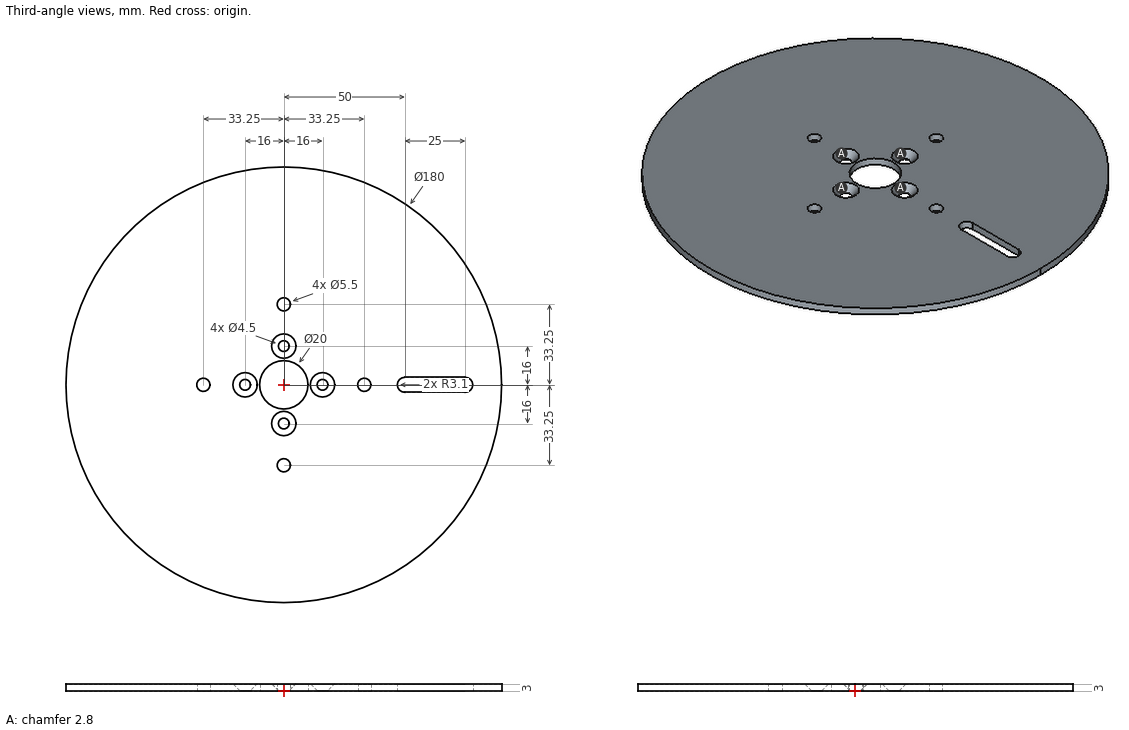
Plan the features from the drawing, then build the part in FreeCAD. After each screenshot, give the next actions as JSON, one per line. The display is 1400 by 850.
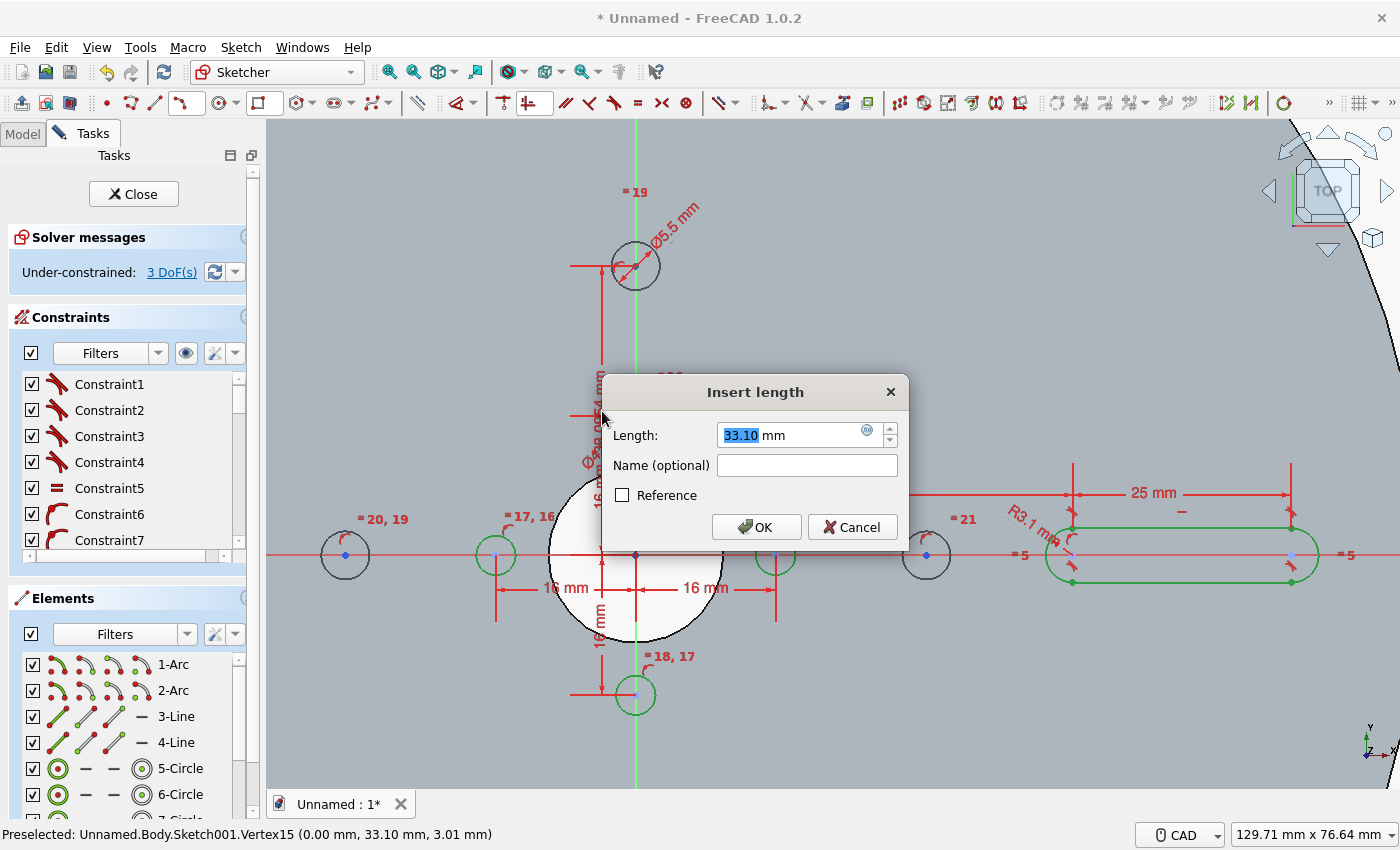
{"action": "type", "text": "33.25"}
{"action": "key", "text": "Return"}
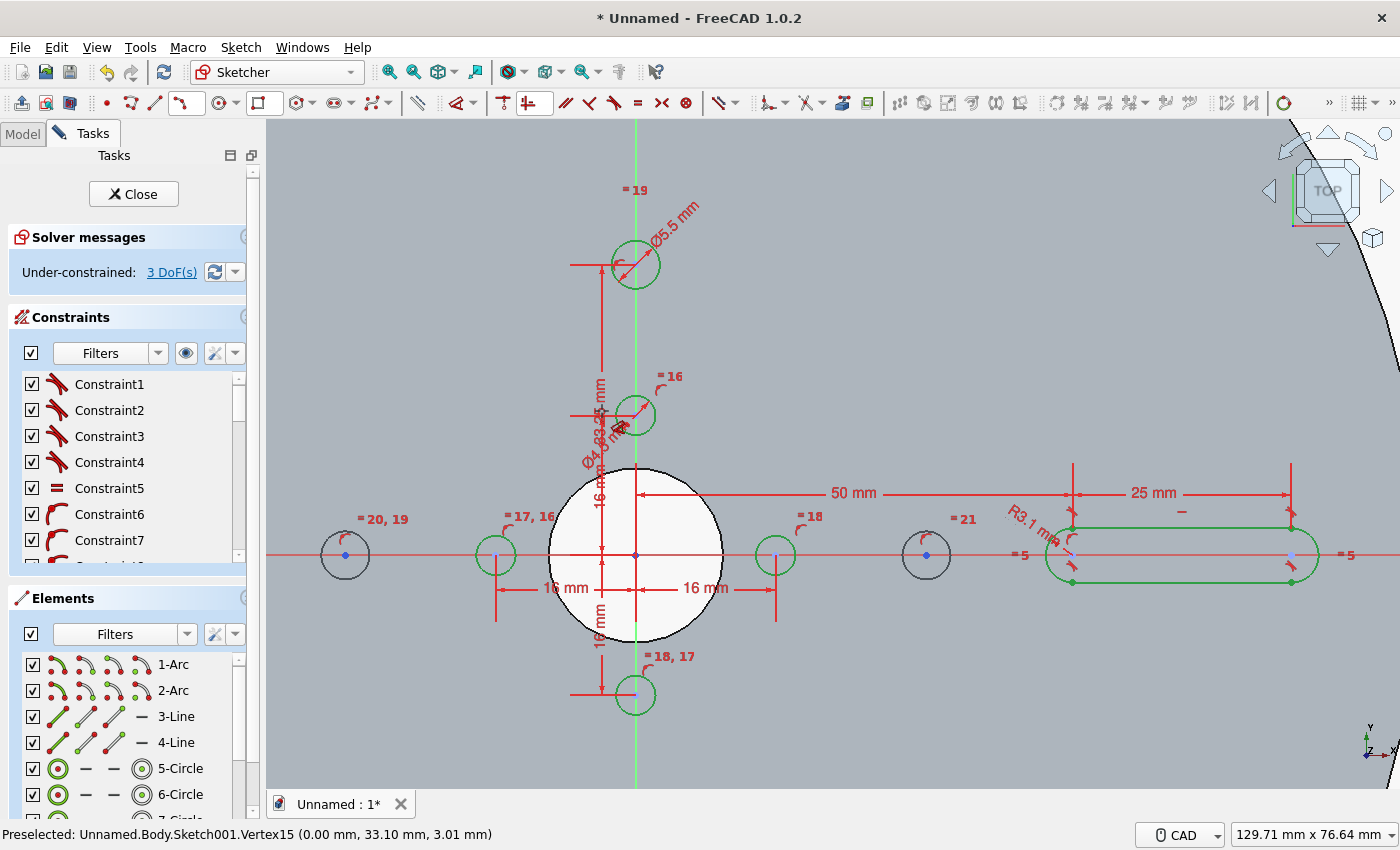
{"action": "left_click", "coordinate": [345, 555]}
{"action": "left_click", "coordinate": [491, 589]}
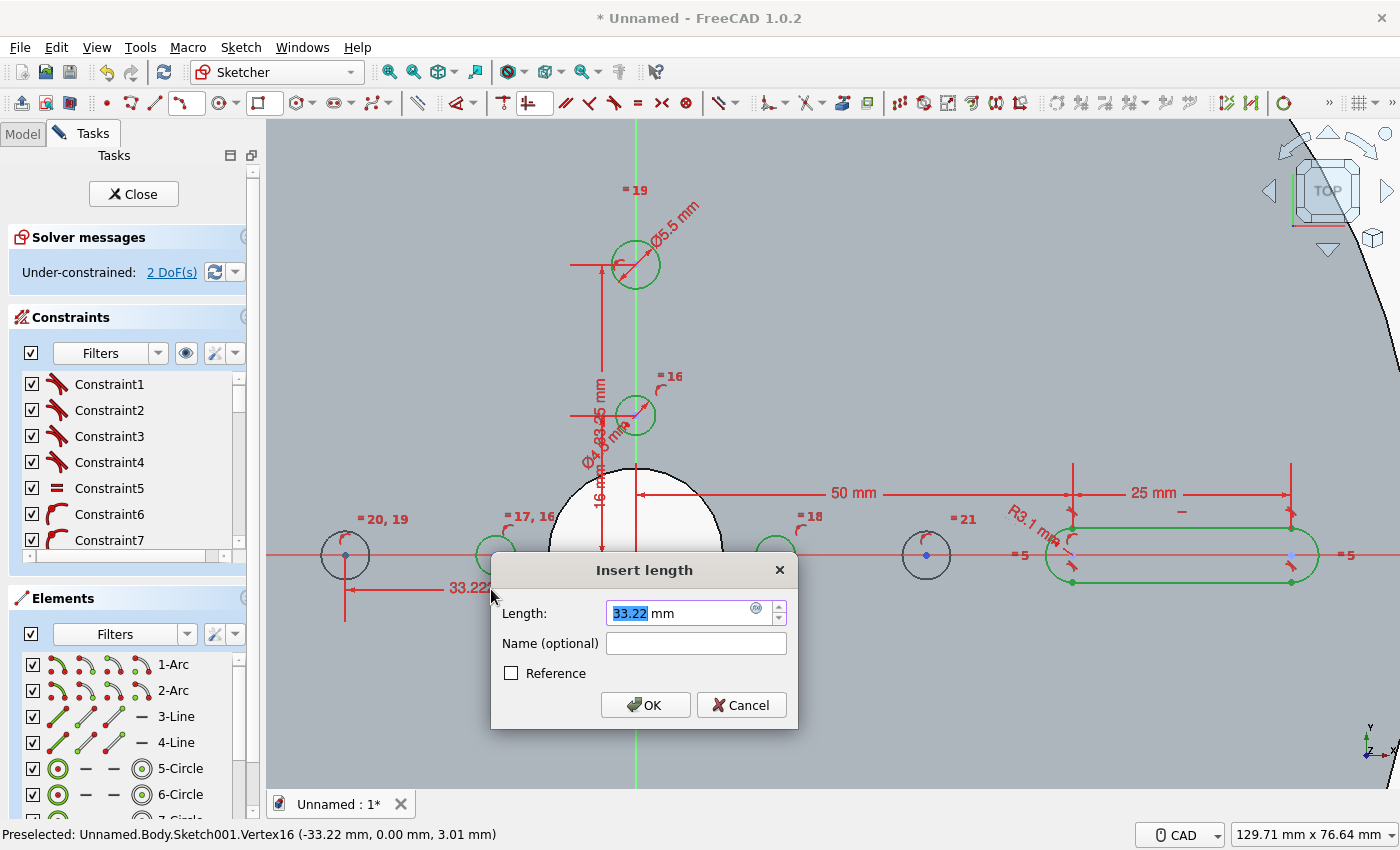
{"action": "type", "text": "33.25"}
{"action": "key", "text": "Return"}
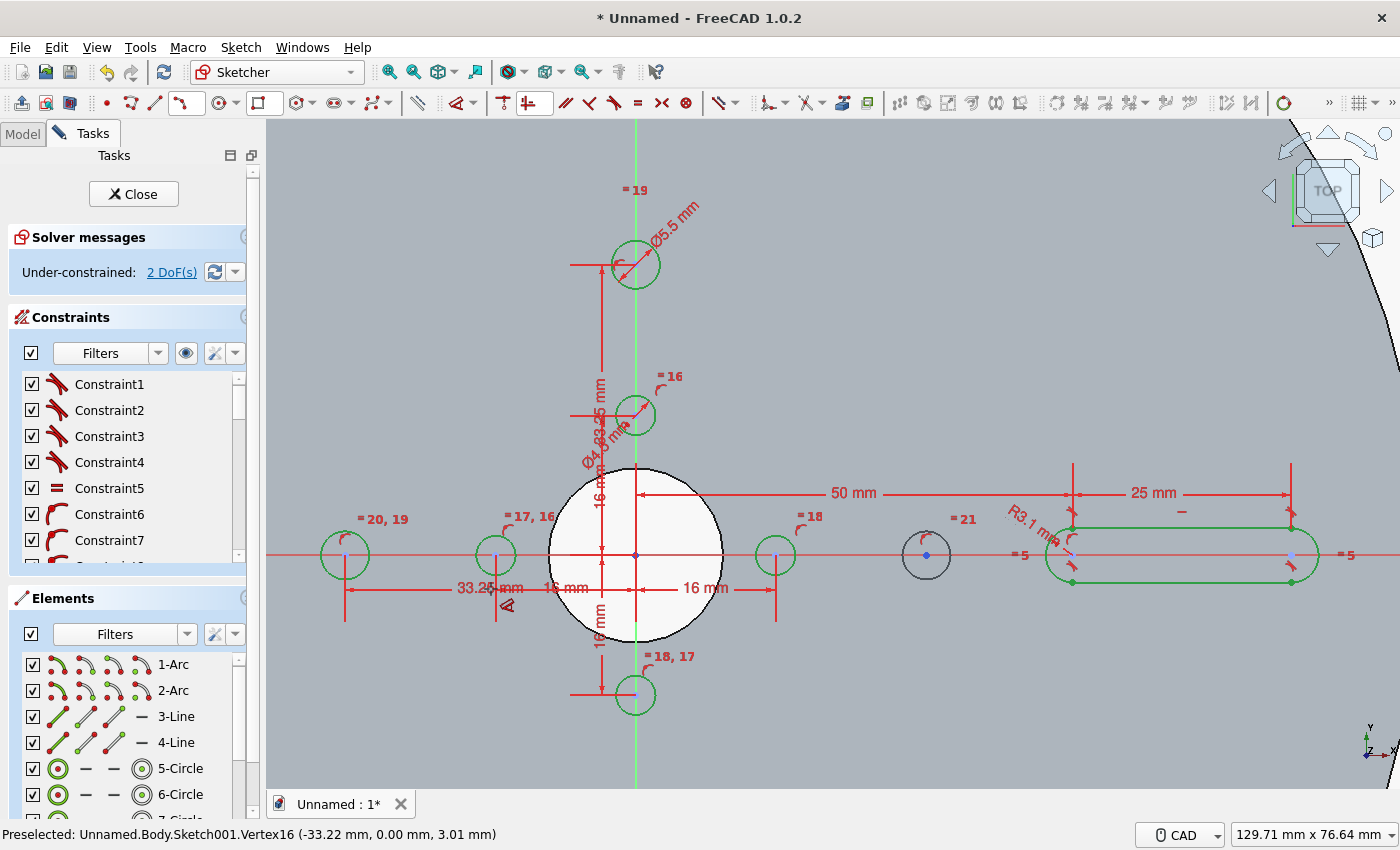
{"action": "scroll", "coordinate": [652, 248], "scroll_direction": "down", "scroll_amount": 2}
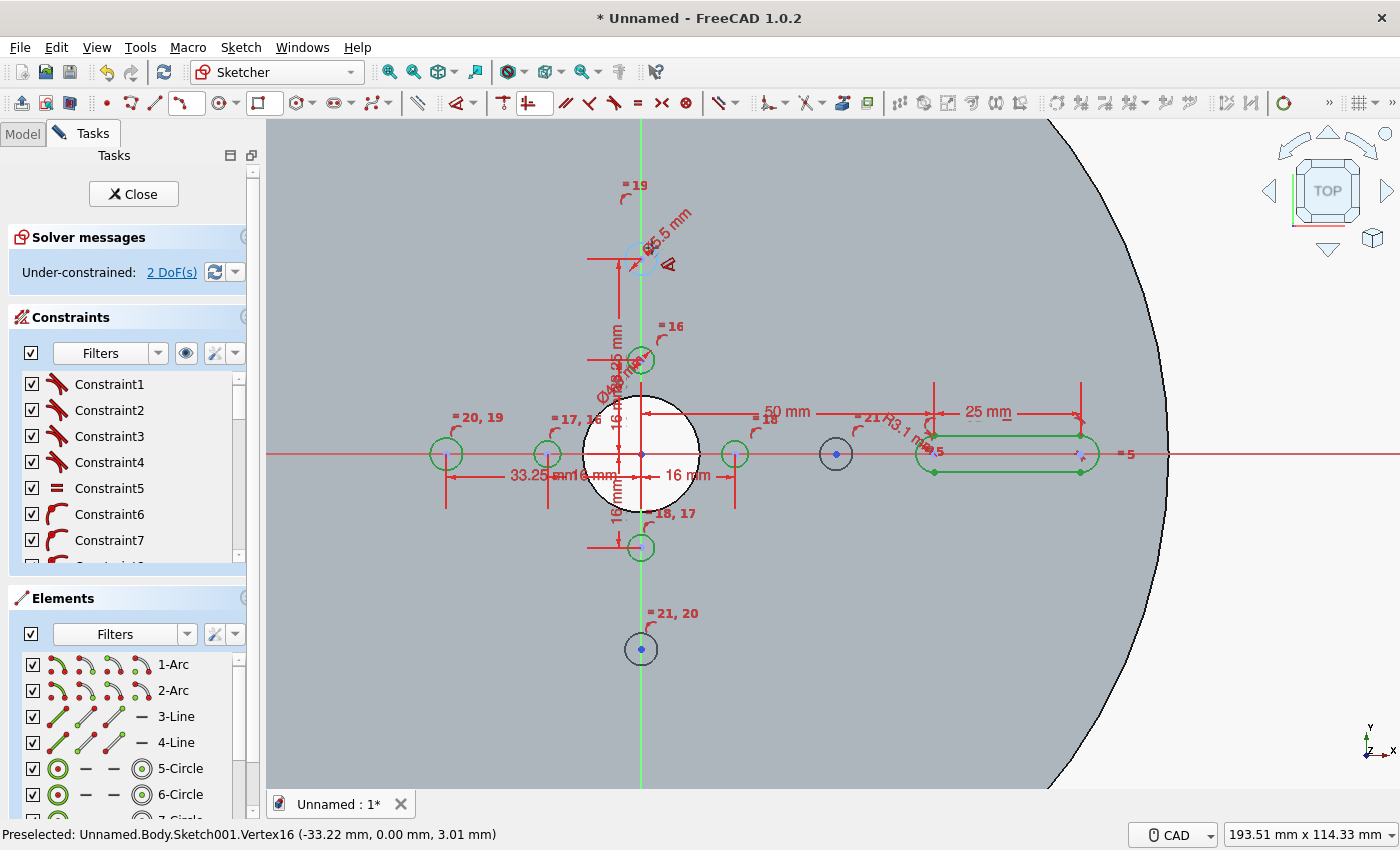
{"action": "left_click", "coordinate": [641, 649]}
{"action": "left_click", "coordinate": [607, 552]}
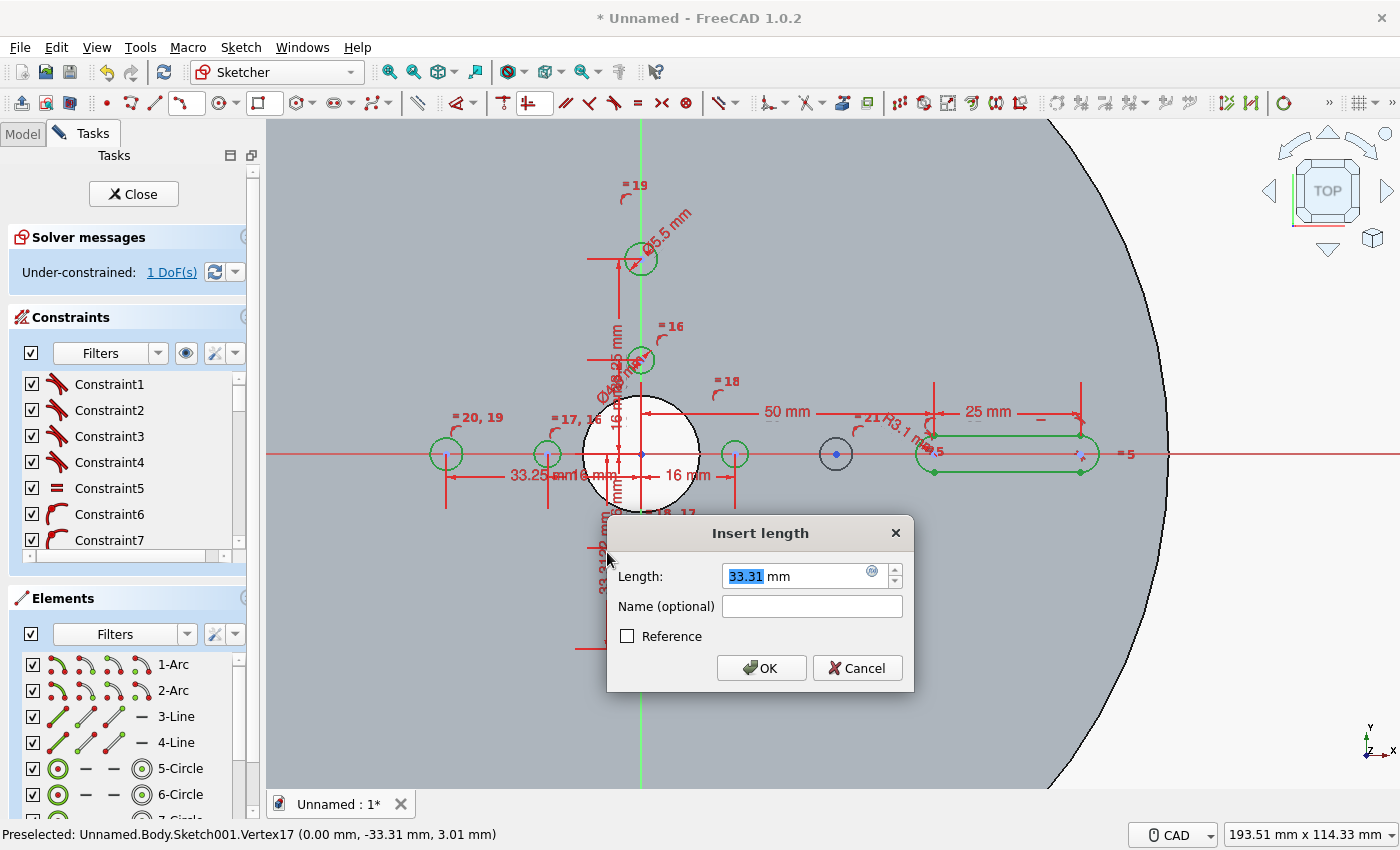
{"action": "type", "text": "33.25"}
{"action": "key", "text": "Return"}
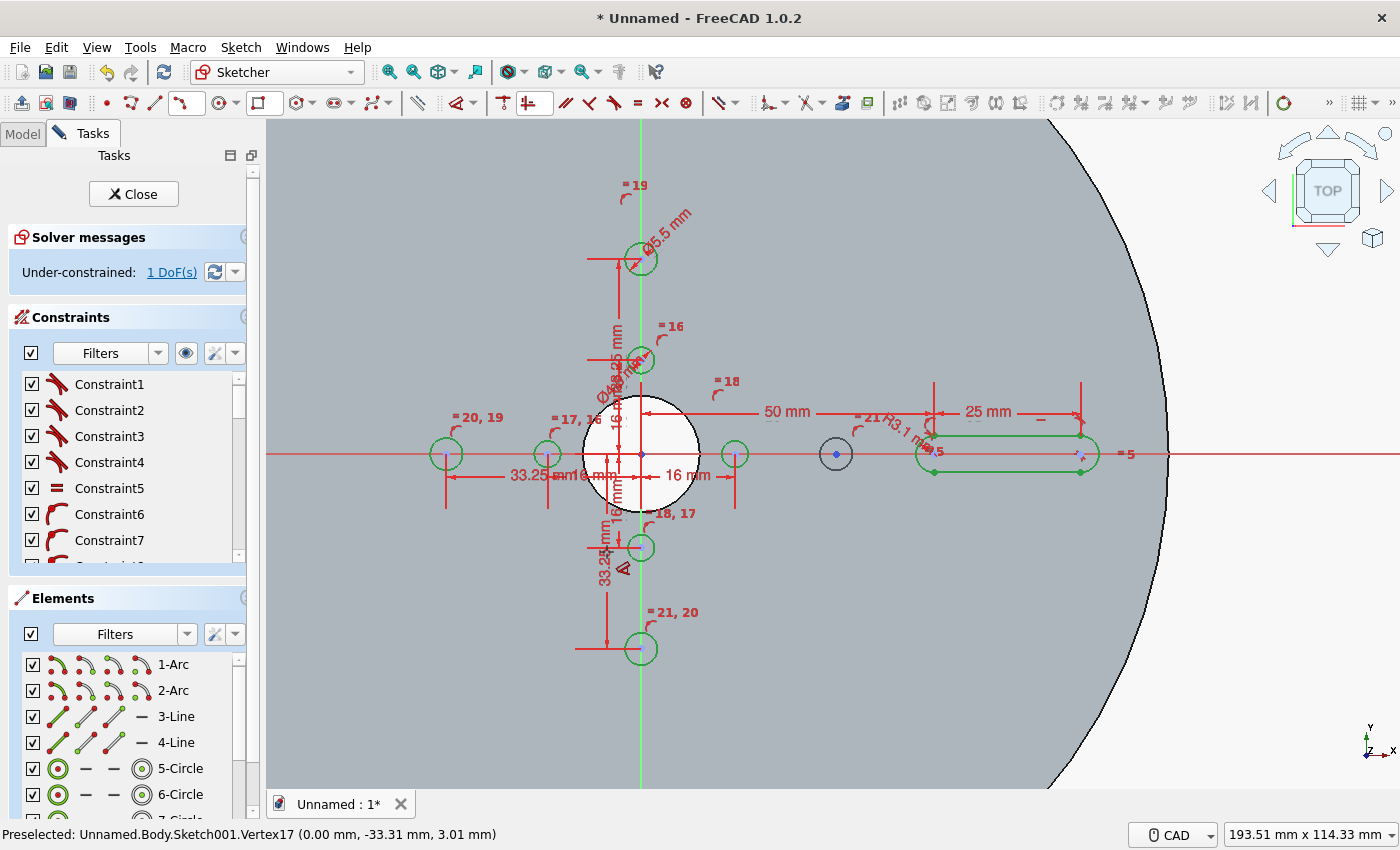
{"action": "left_click", "coordinate": [836, 454]}
{"action": "left_click", "coordinate": [783, 488]}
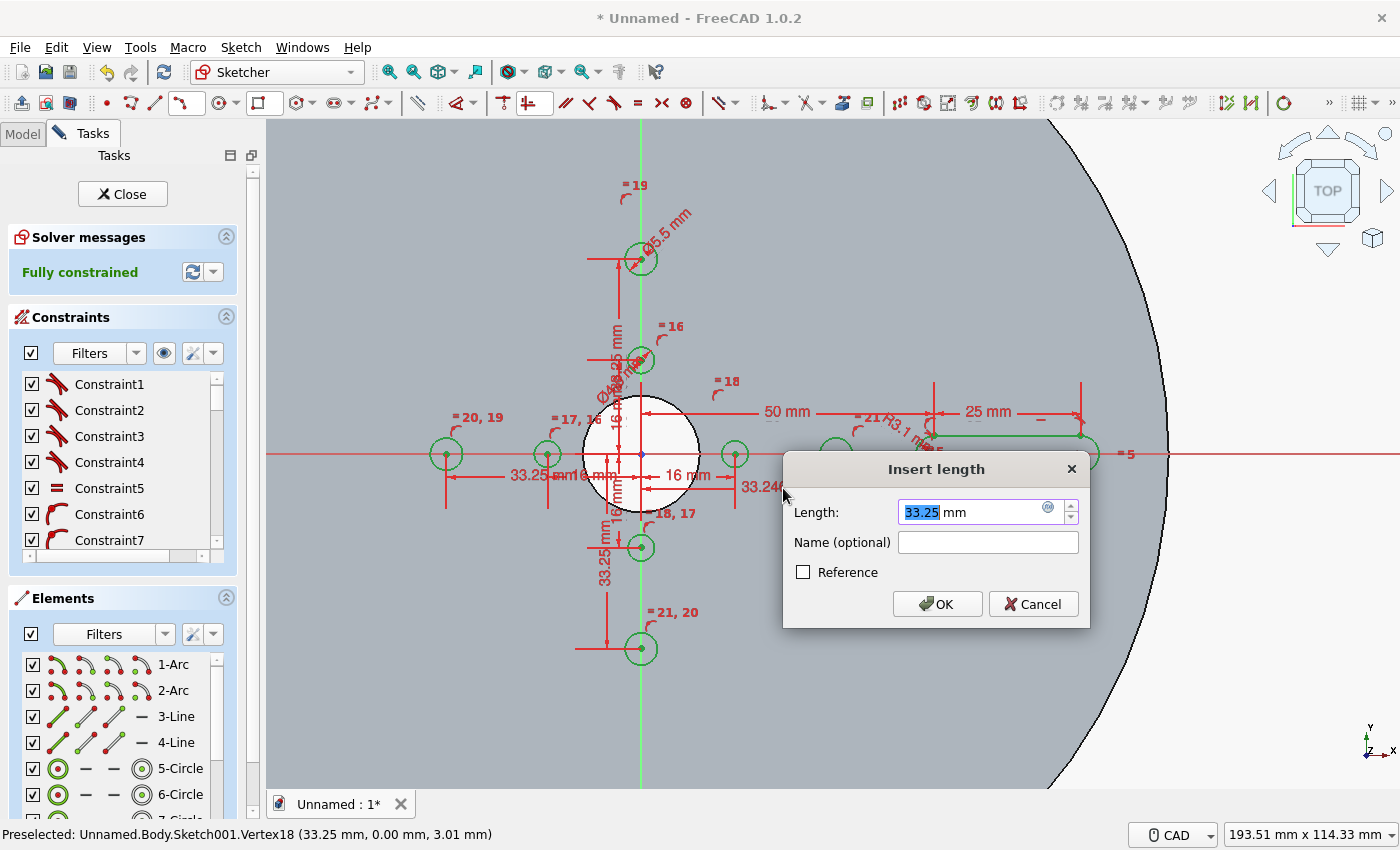
{"action": "type", "text": "33.25"}
{"action": "key", "text": "Return"}
{"action": "key", "text": "Escape"}